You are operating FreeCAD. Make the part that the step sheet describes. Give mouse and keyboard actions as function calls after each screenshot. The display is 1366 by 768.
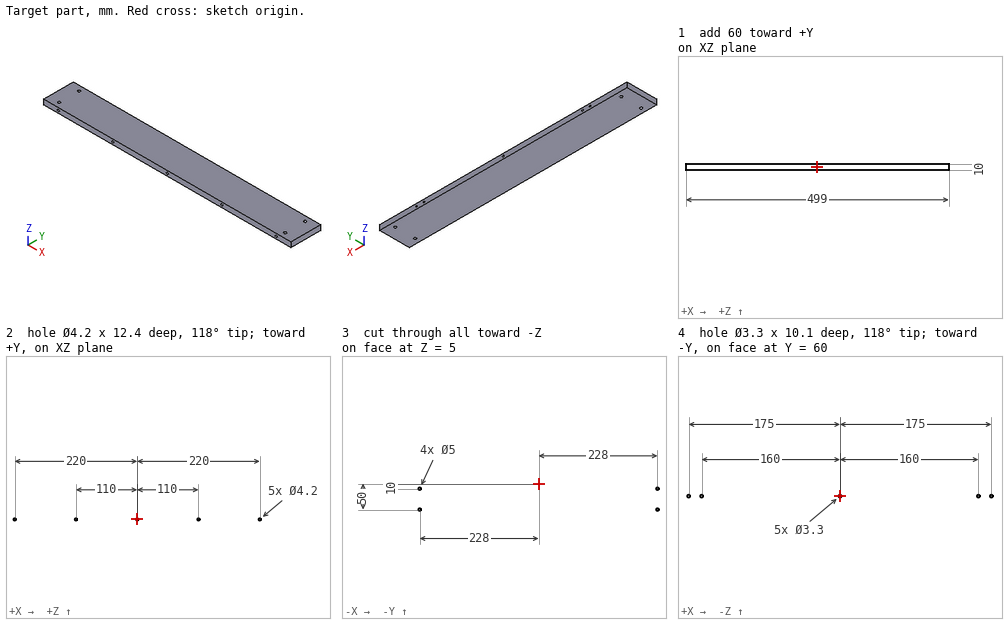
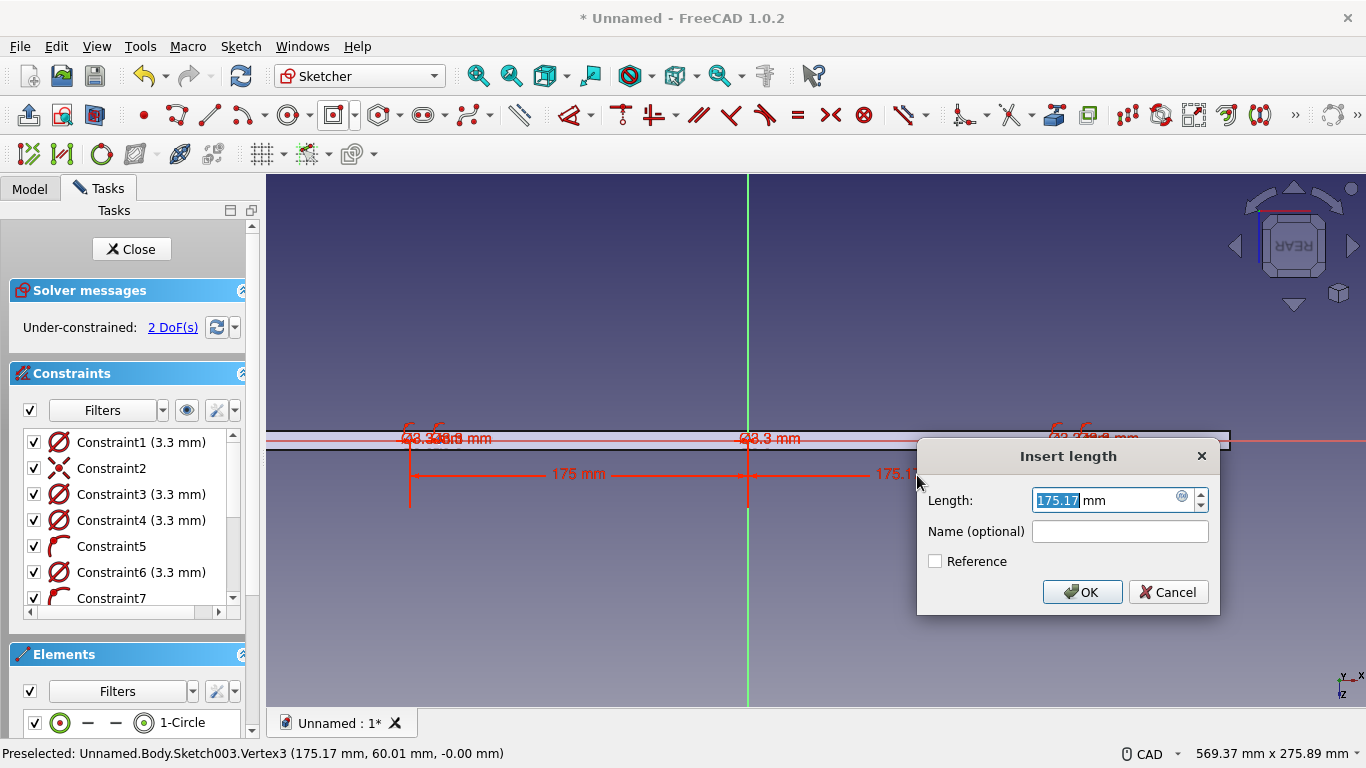
text(175)
key(Return)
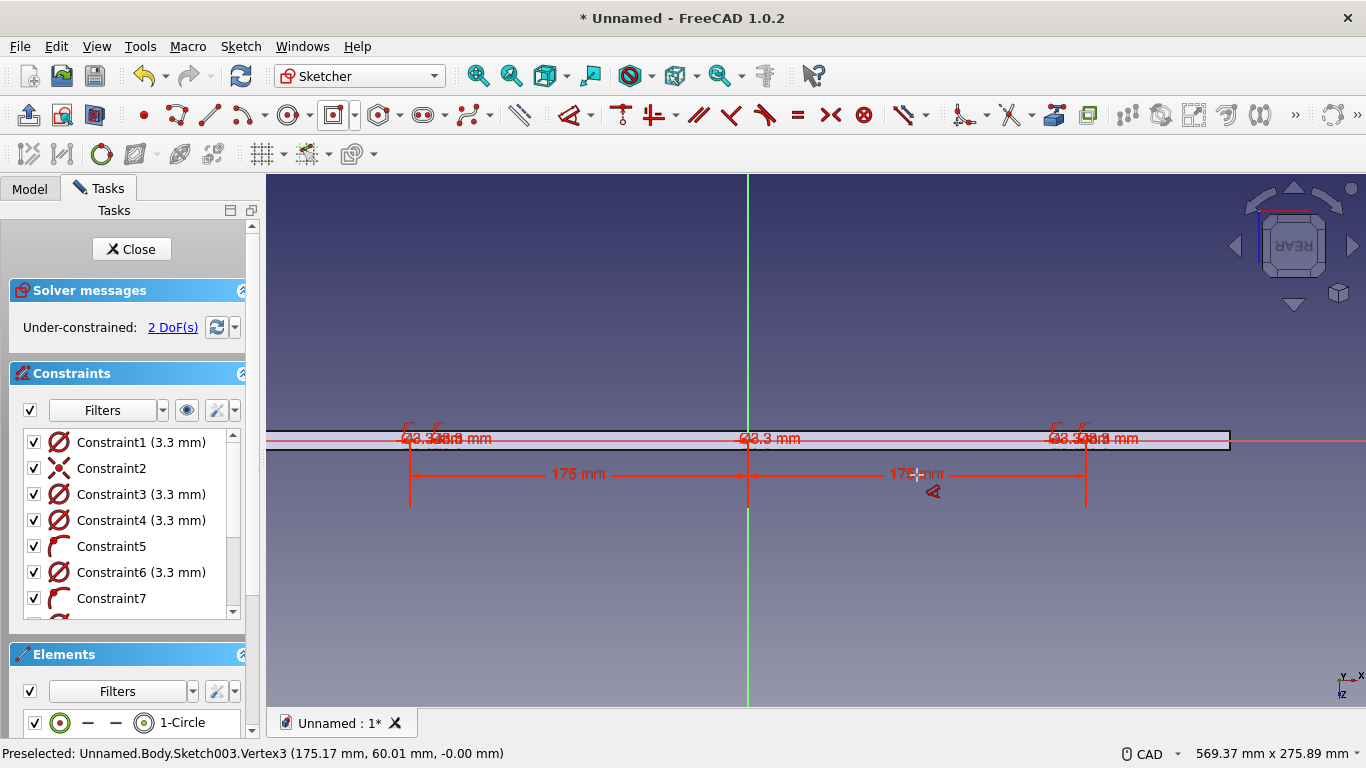
click(439, 441)
click(664, 475)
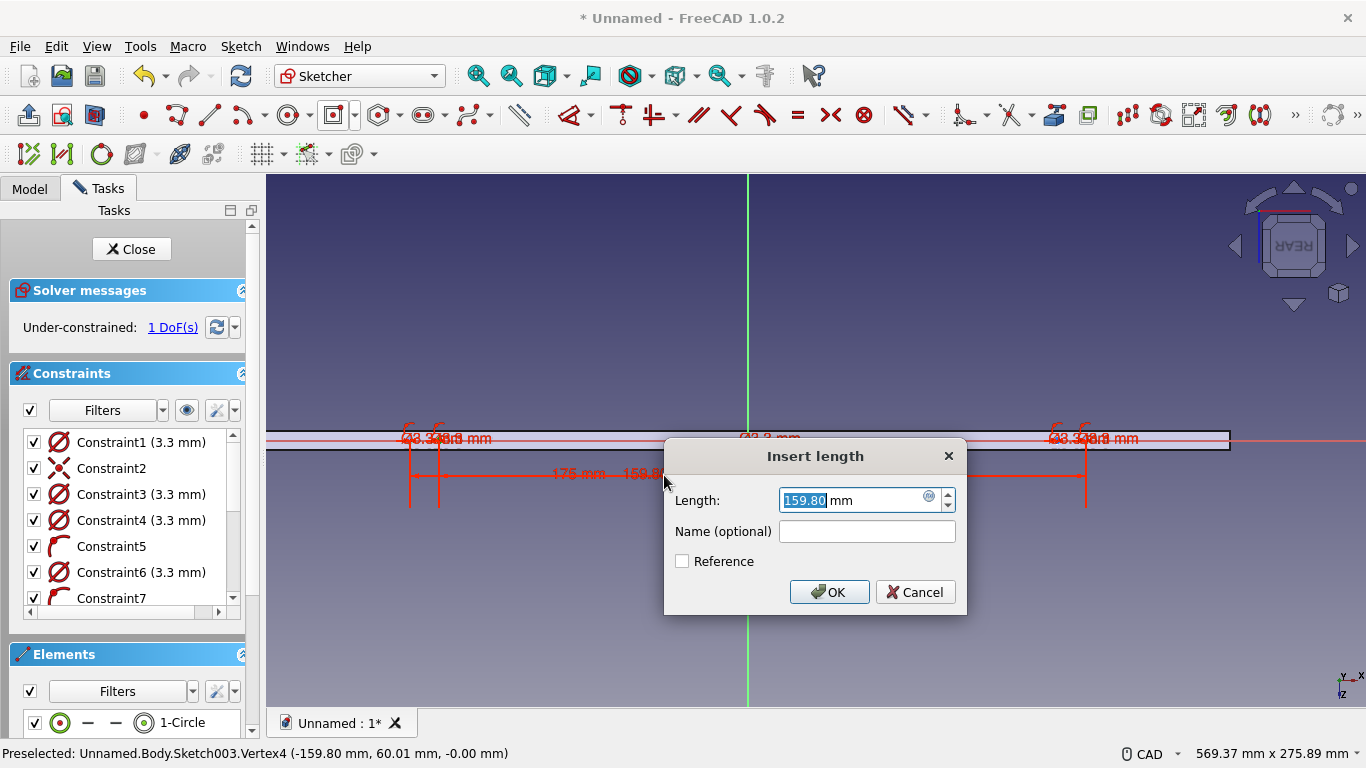
text(160)
key(Return)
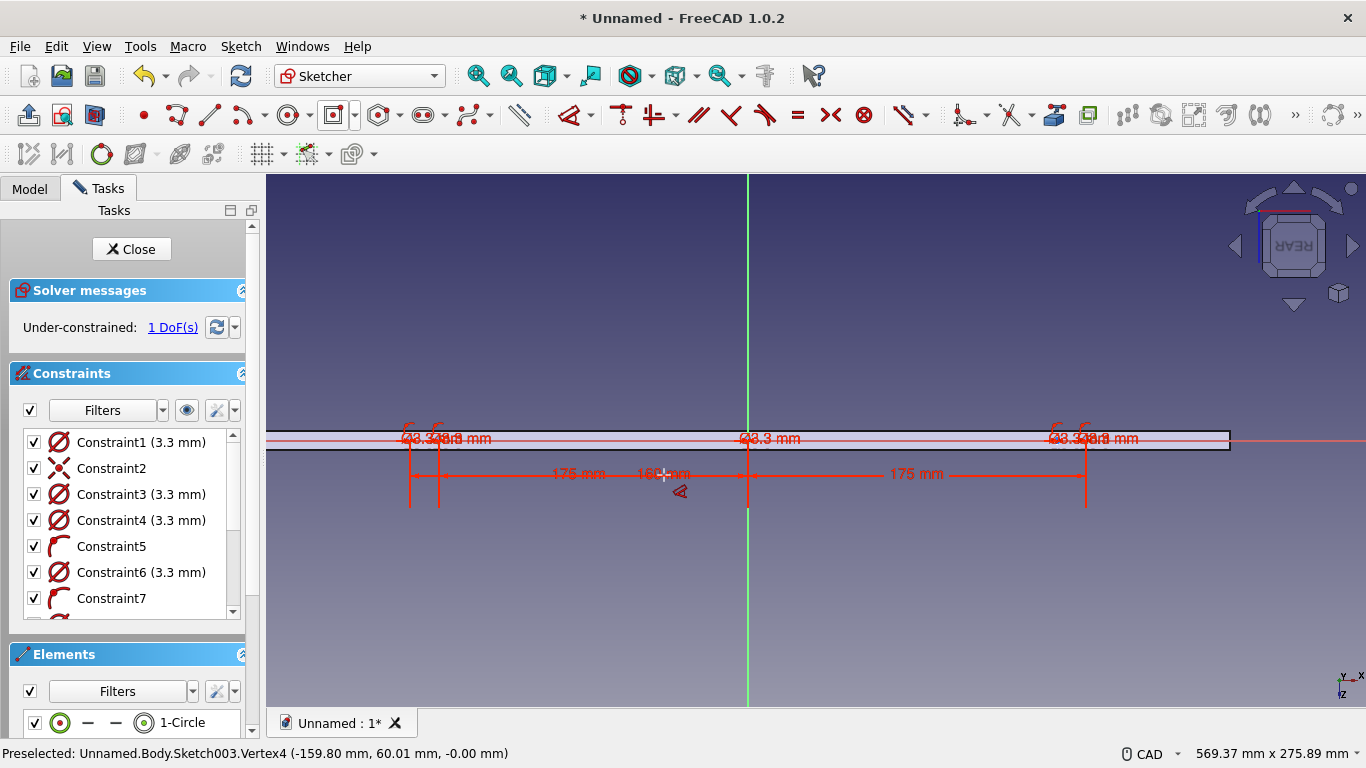
click(1057, 441)
click(831, 475)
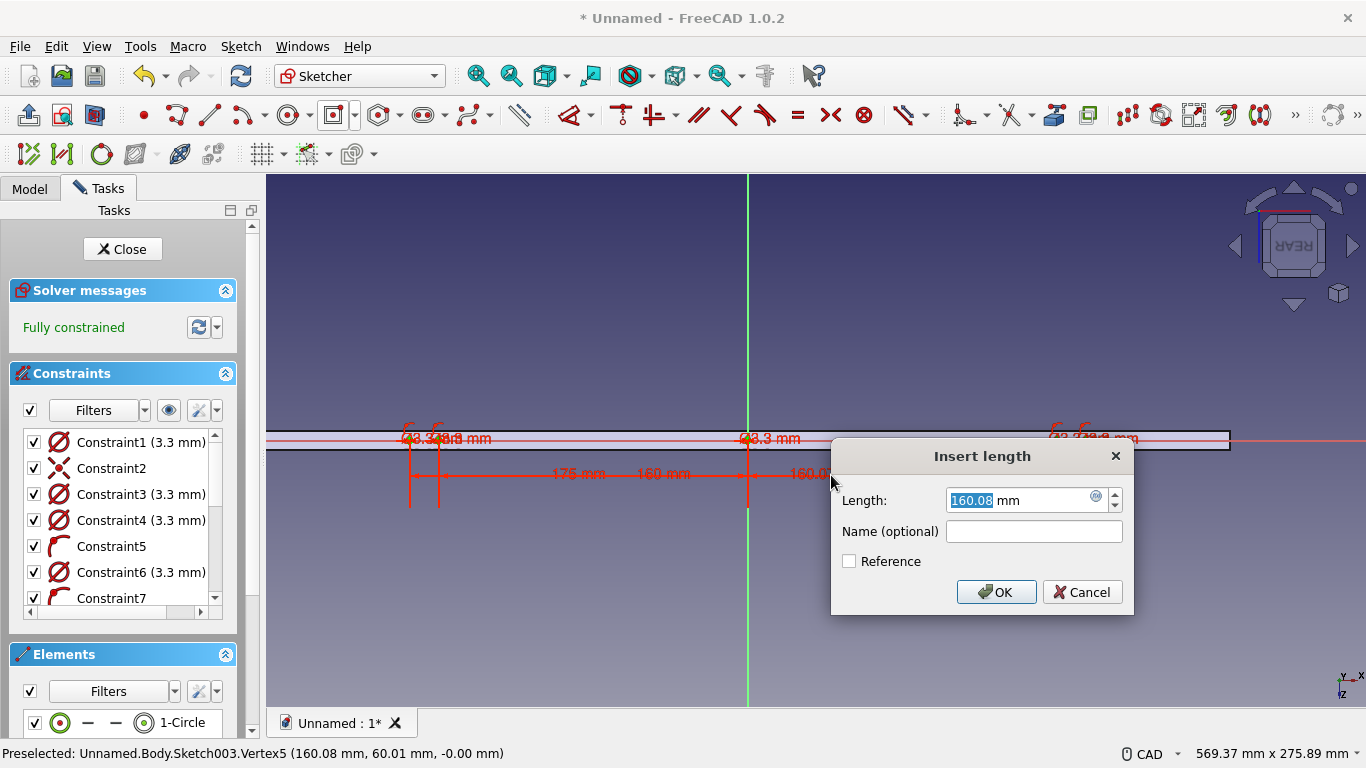
text(160)
key(Return)
key(Escape)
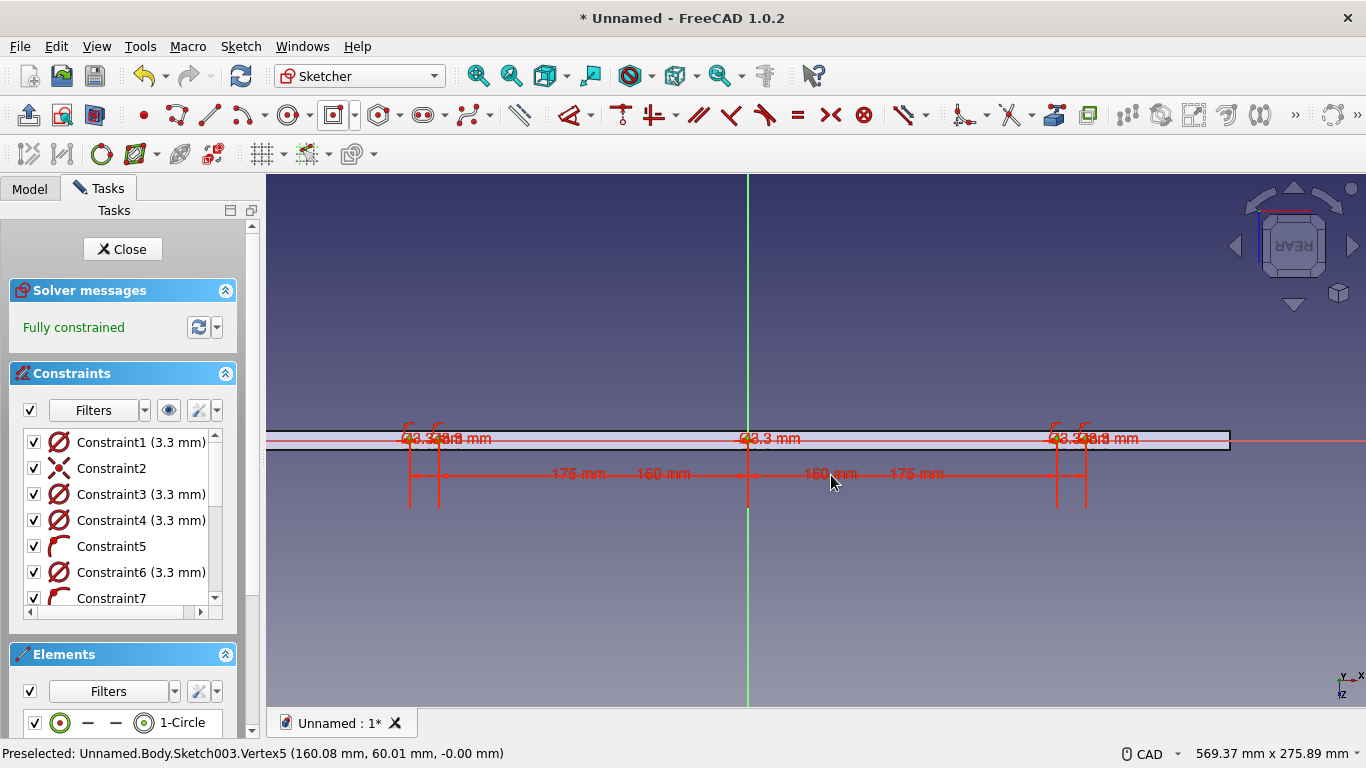
click(123, 249)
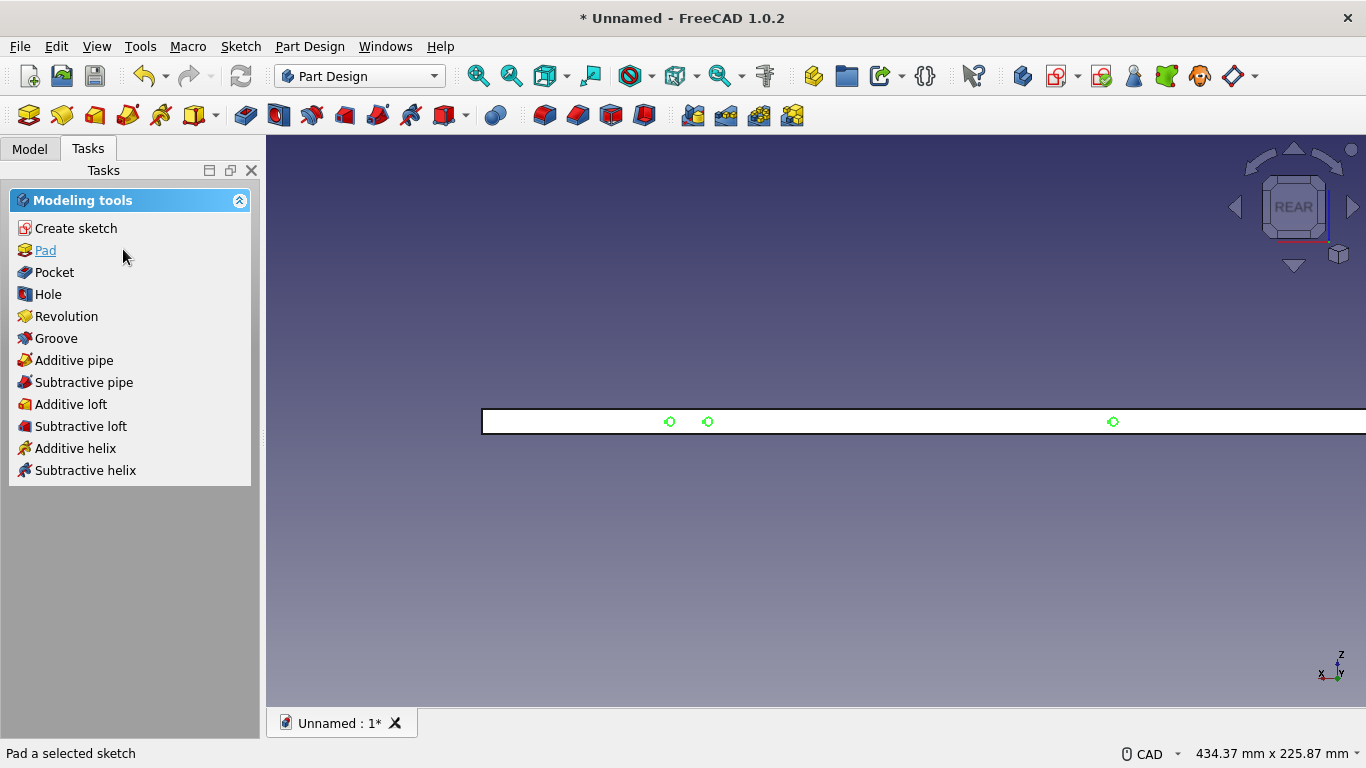
click(279, 116)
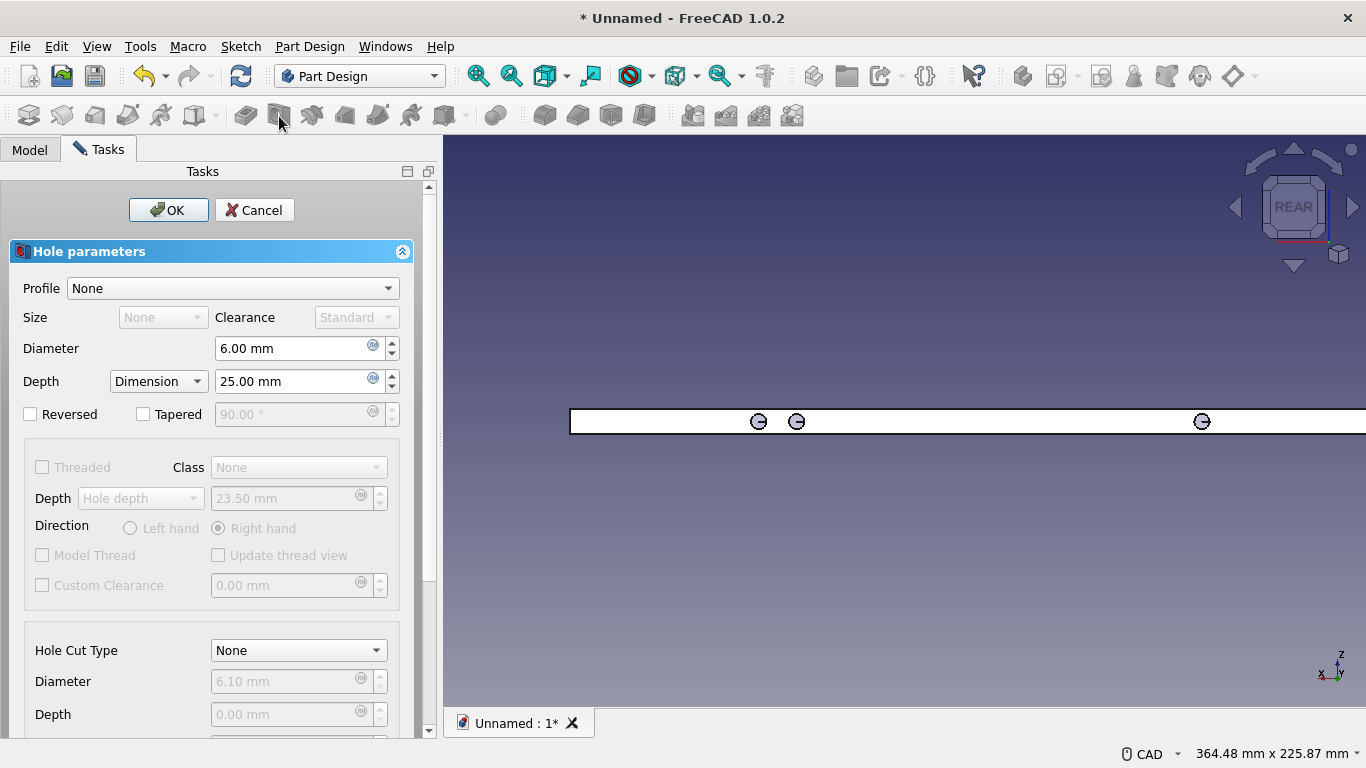
triple_click(300, 348)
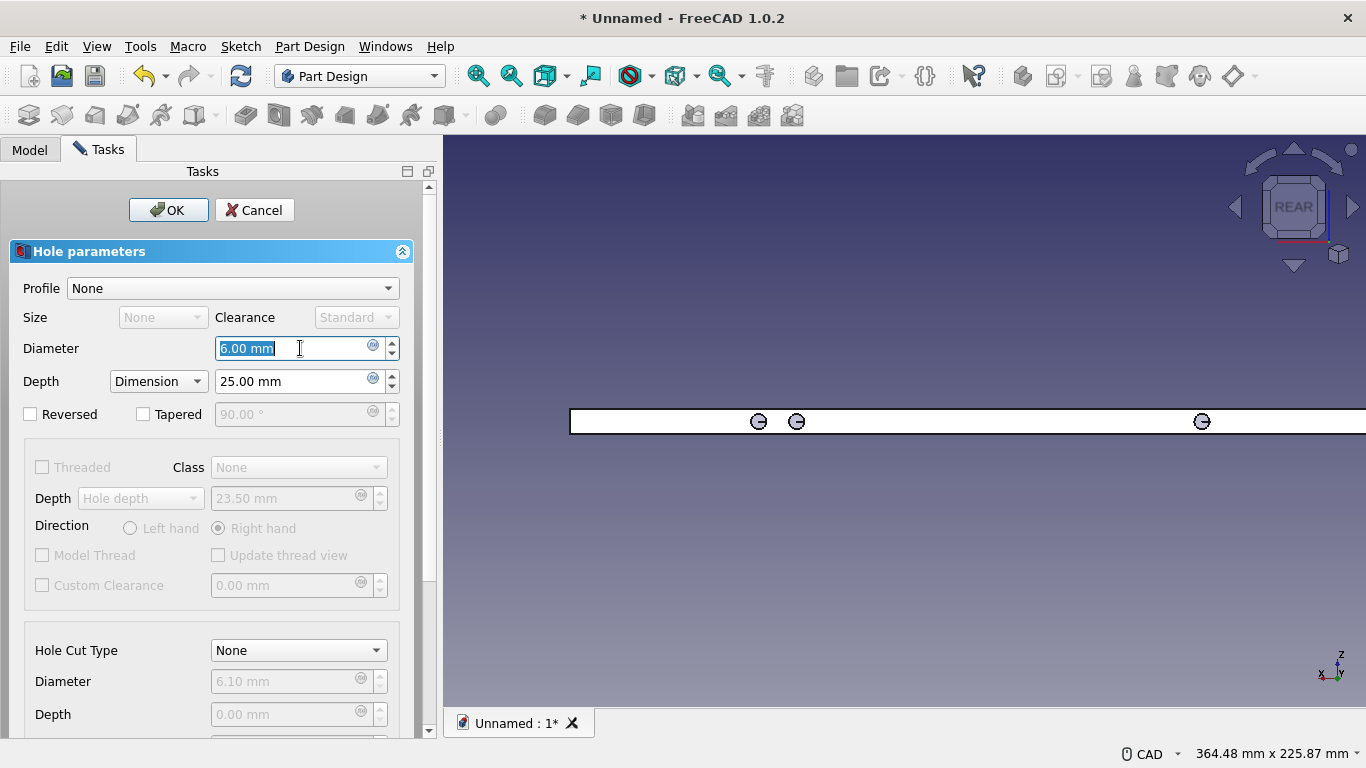
text(3.3)
key(Tab)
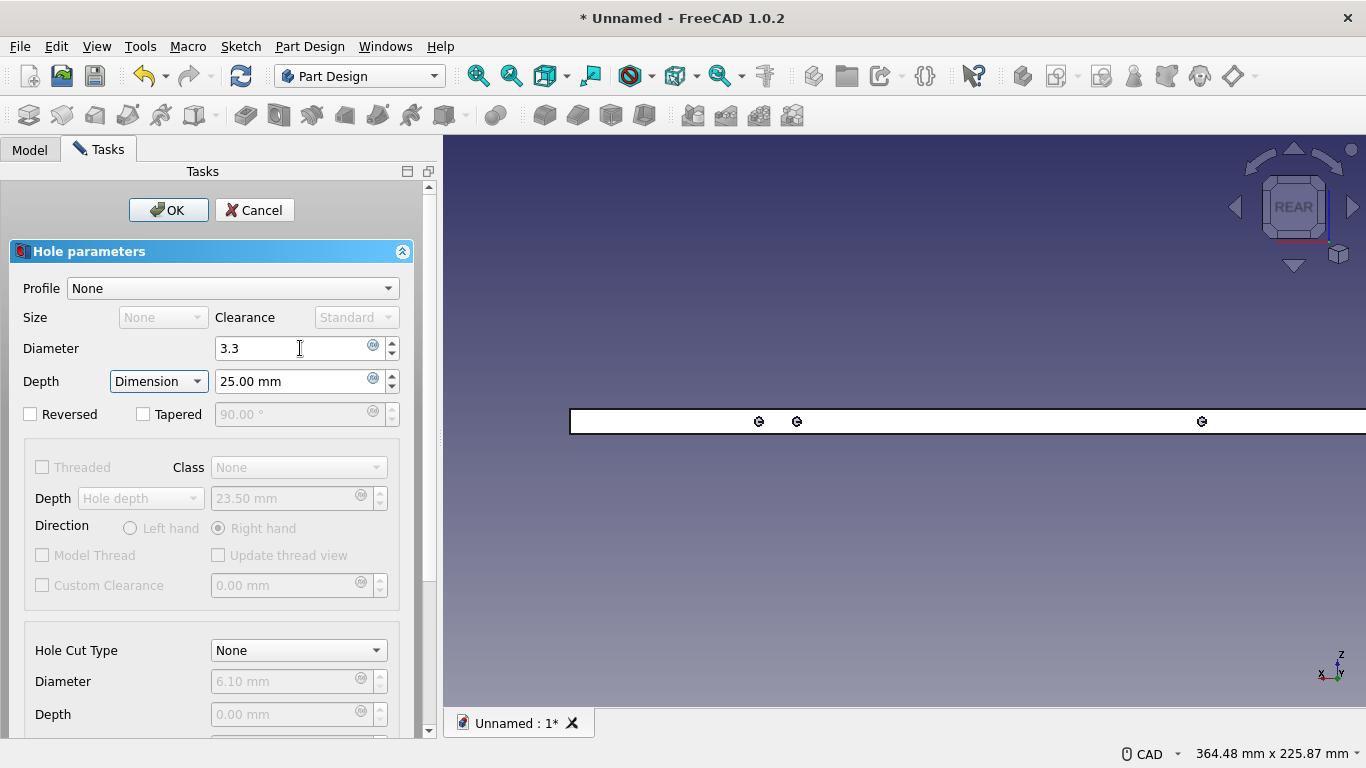
triple_click(300, 382)